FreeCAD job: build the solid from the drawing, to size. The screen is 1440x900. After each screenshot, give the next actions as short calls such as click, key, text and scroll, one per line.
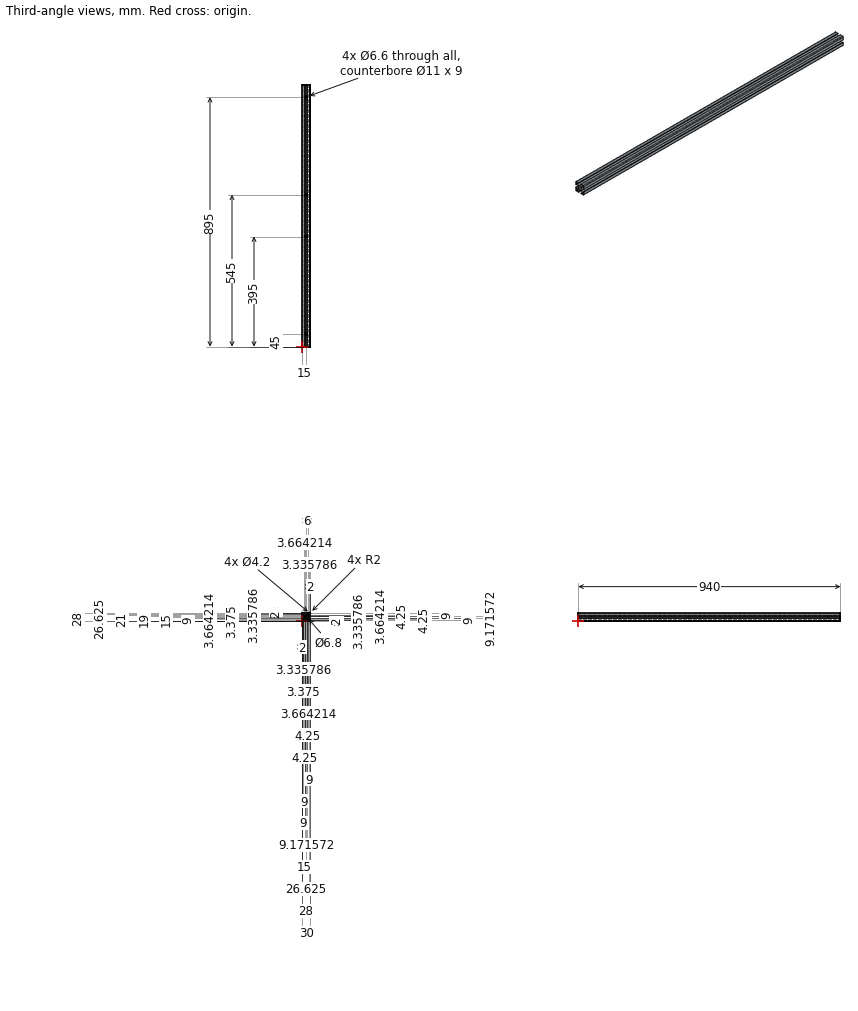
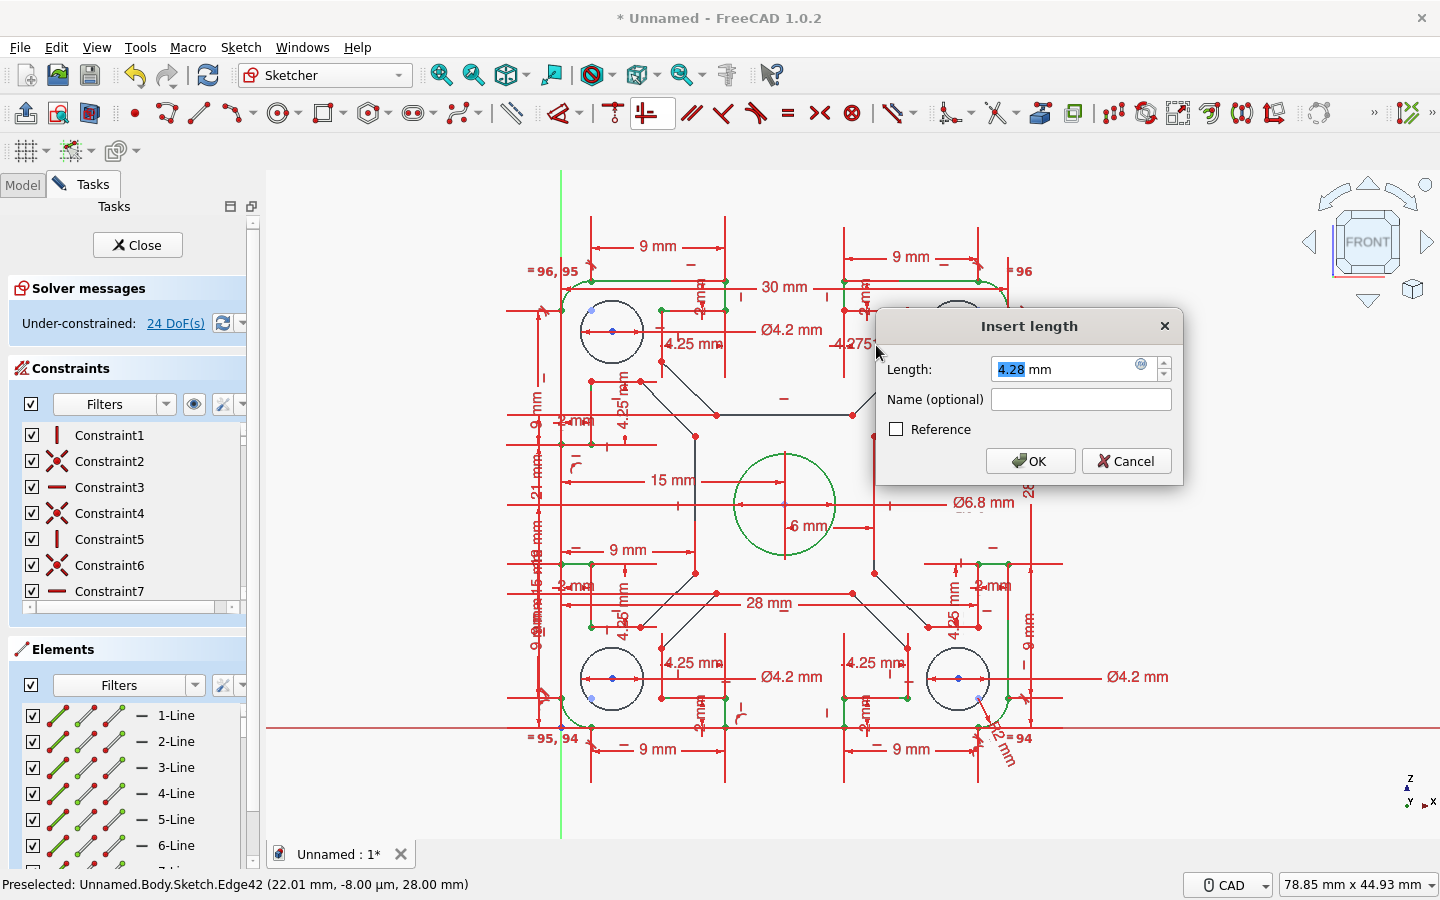
text(4.25)
key(Return)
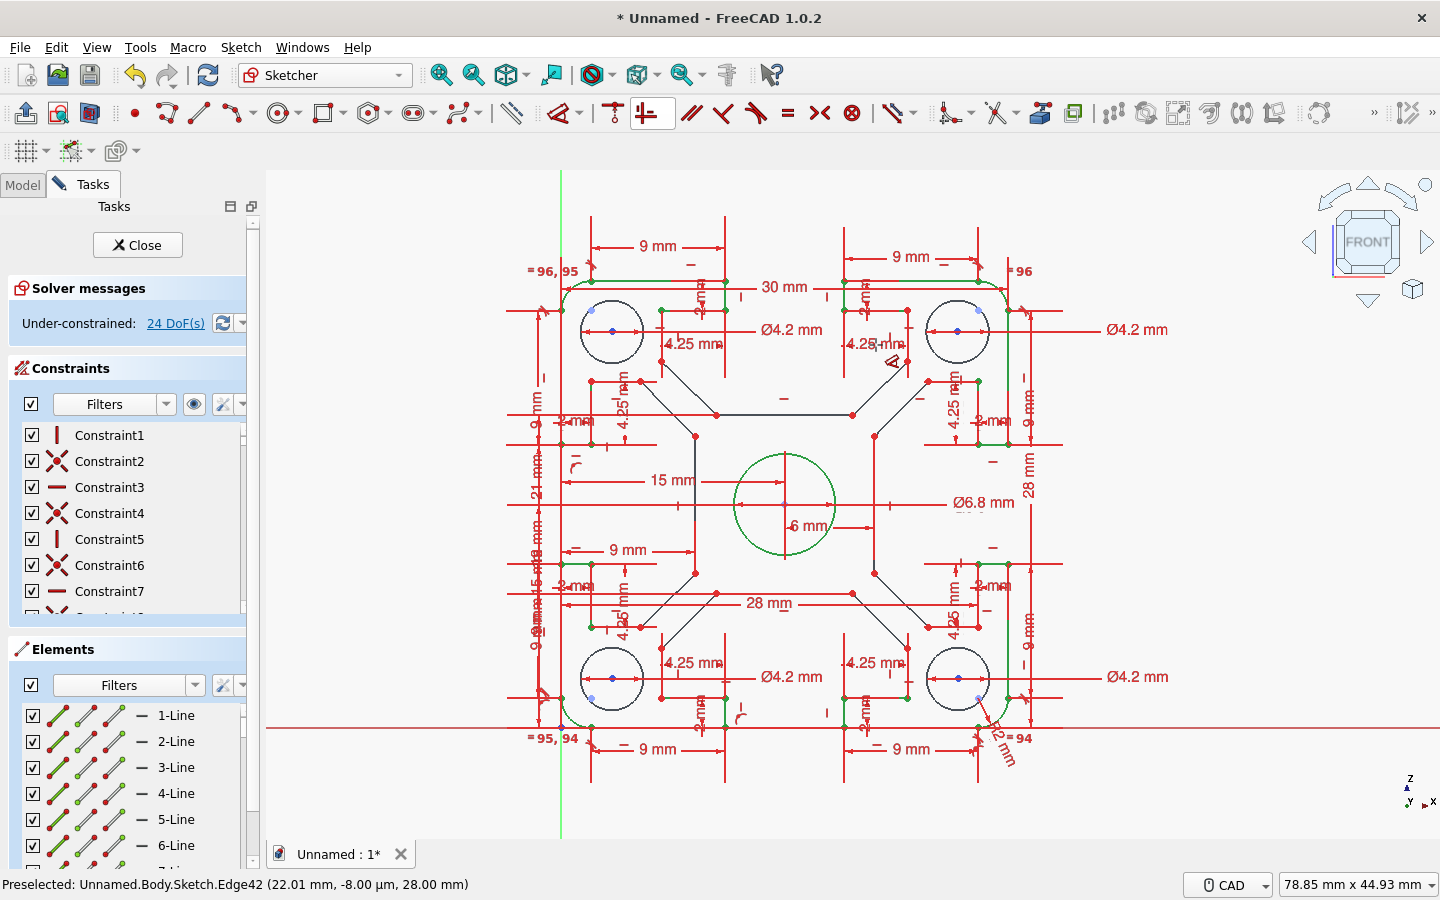
click(612, 332)
click(587, 762)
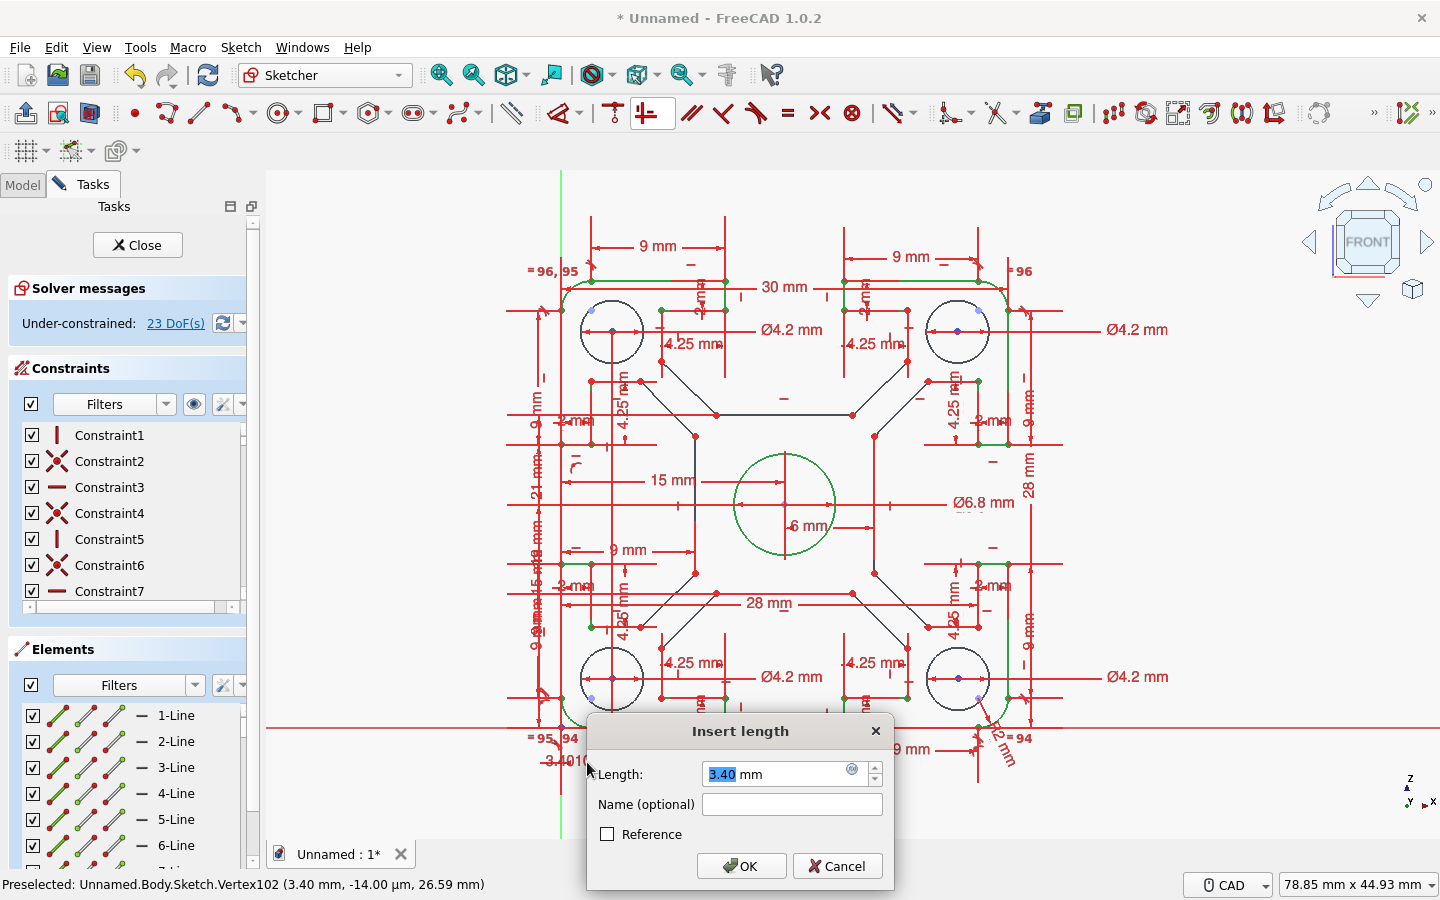
text(3.375)
key(Return)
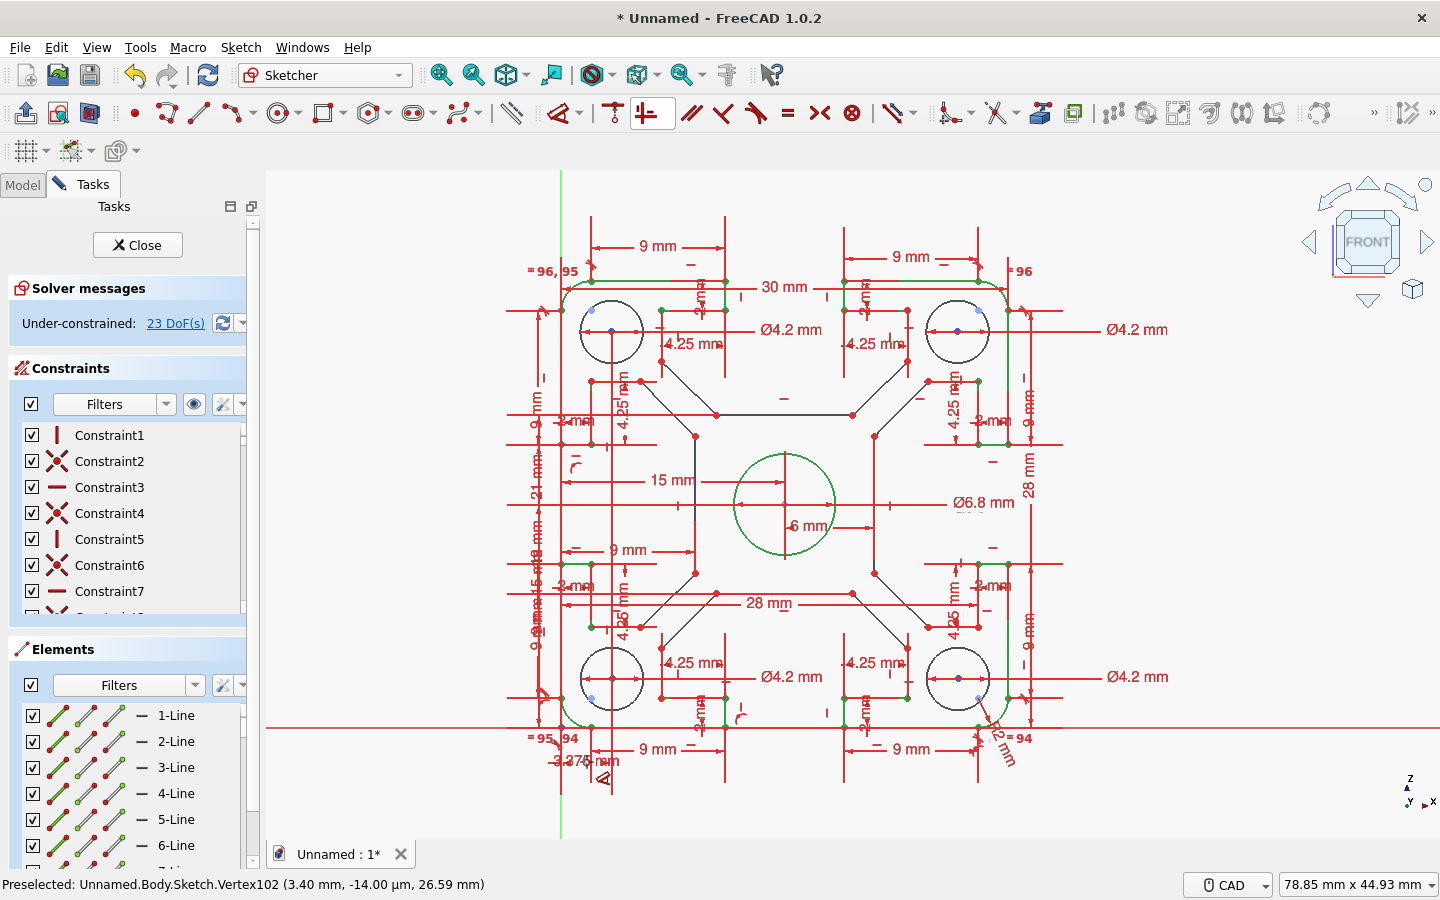
click(958, 679)
click(527, 703)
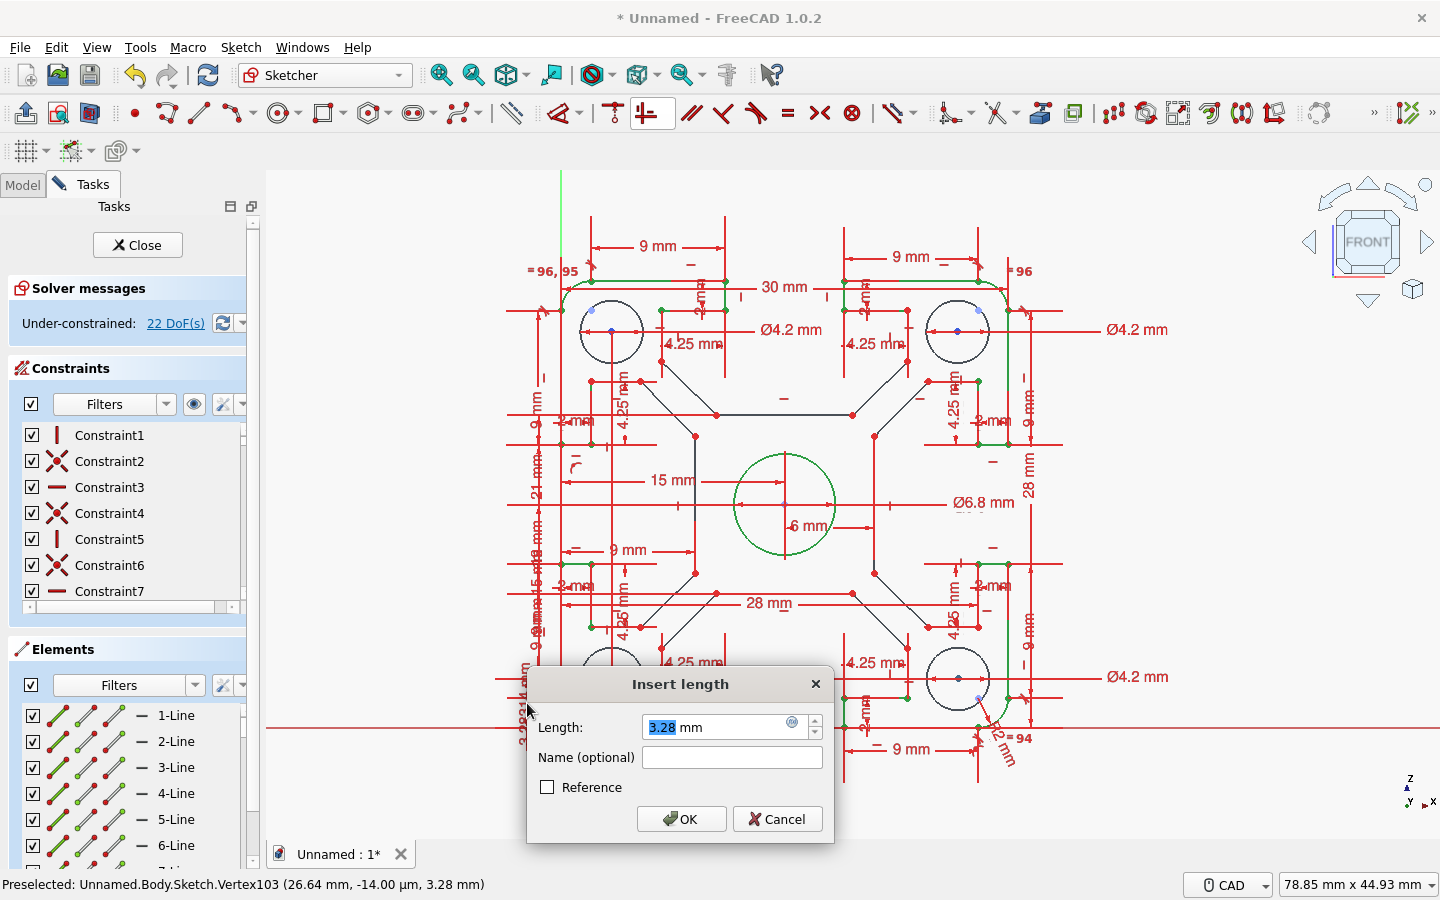
text(3.375)
key(Return)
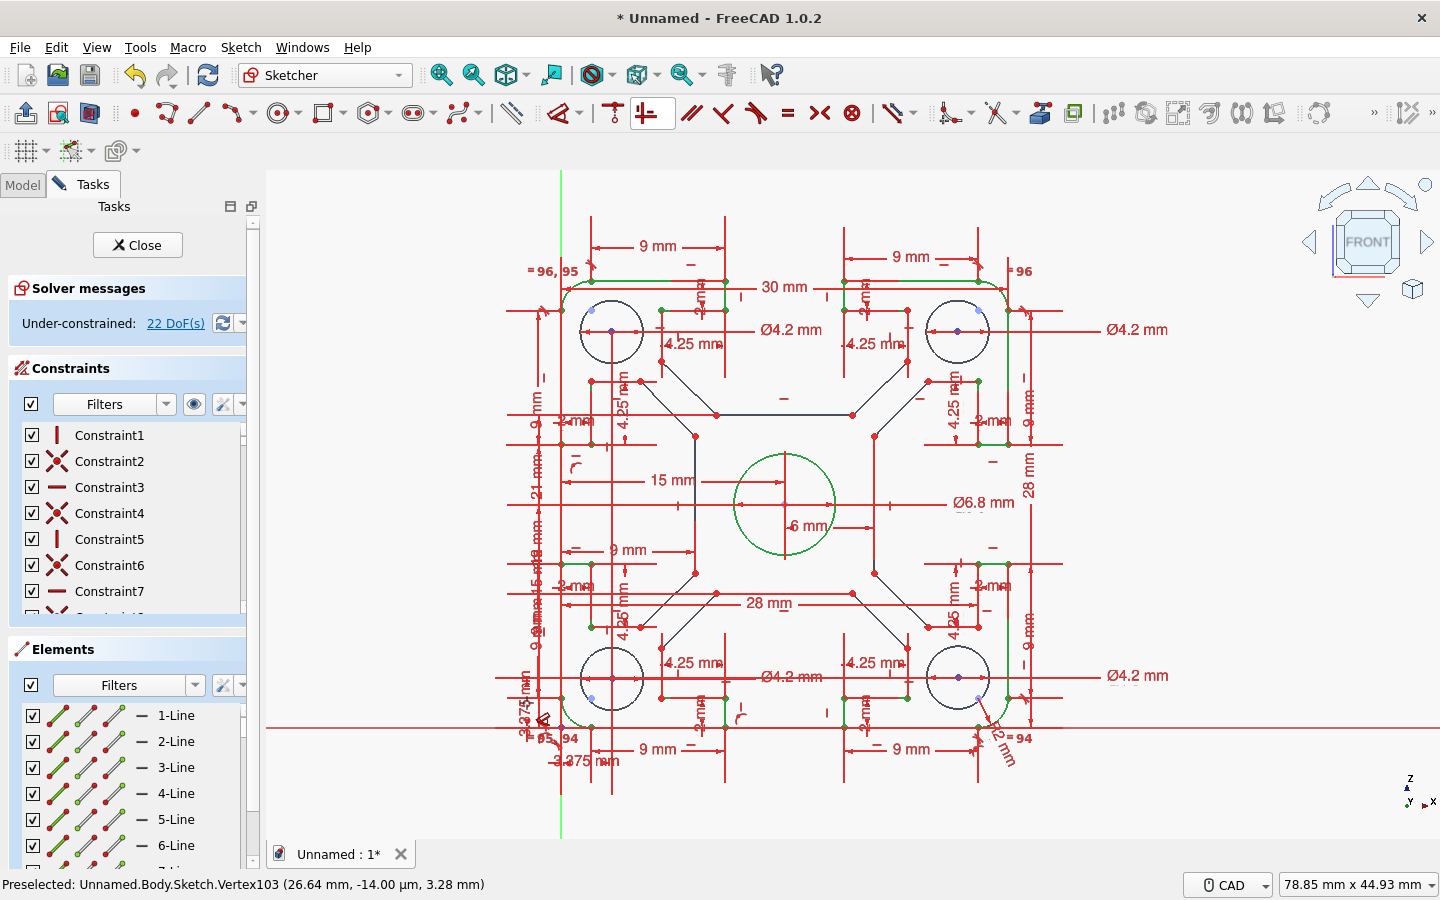
click(612, 679)
click(587, 786)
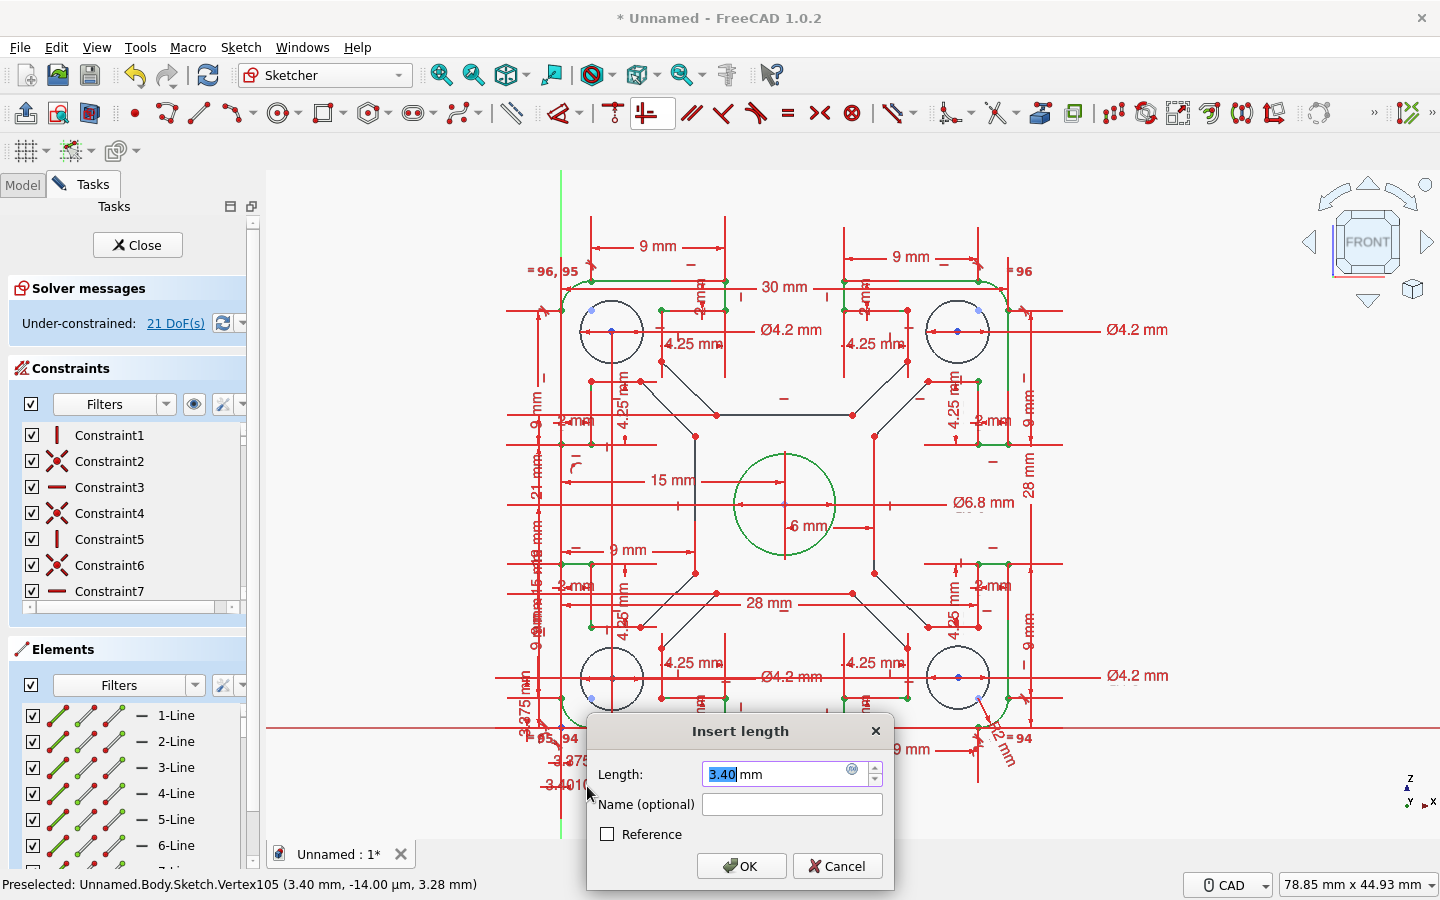
text(3.375)
key(Return)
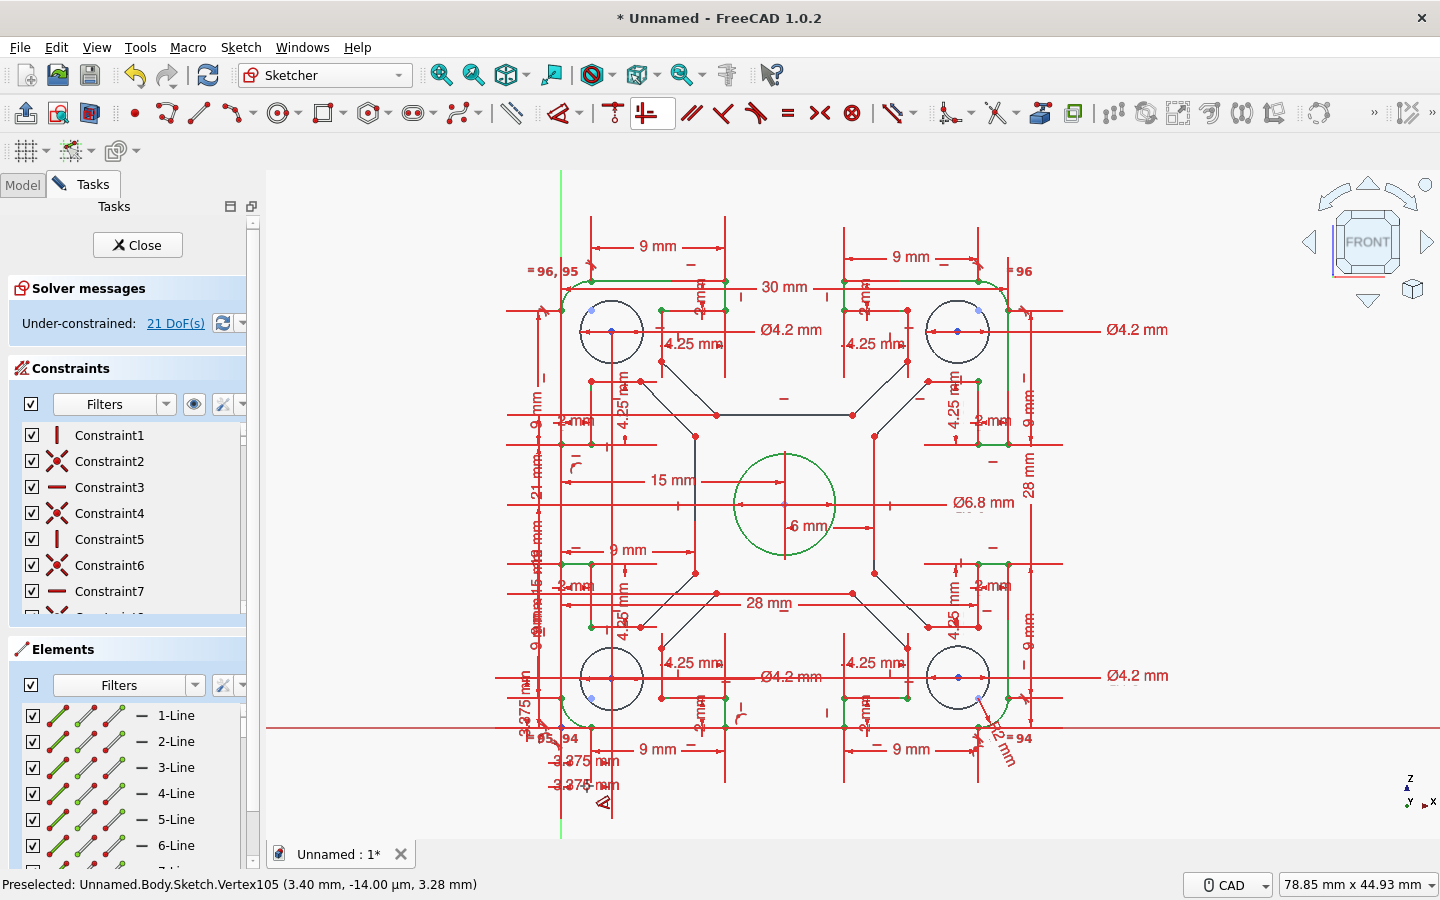
click(612, 679)
click(455, 703)